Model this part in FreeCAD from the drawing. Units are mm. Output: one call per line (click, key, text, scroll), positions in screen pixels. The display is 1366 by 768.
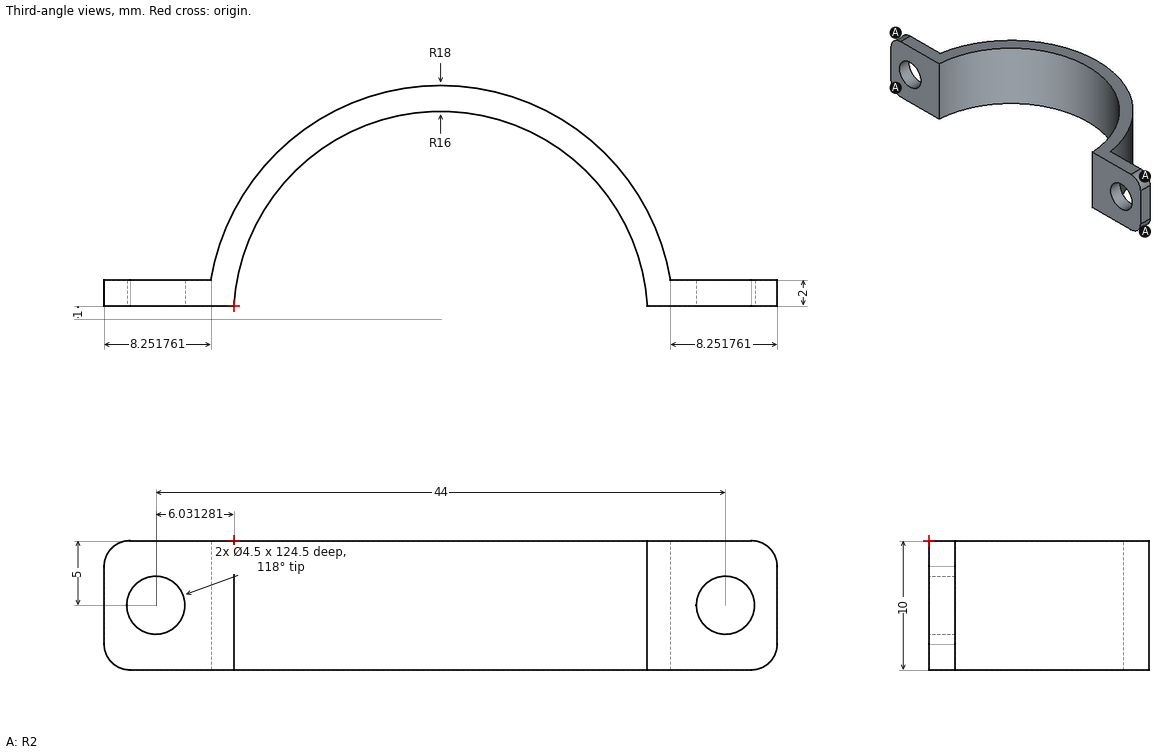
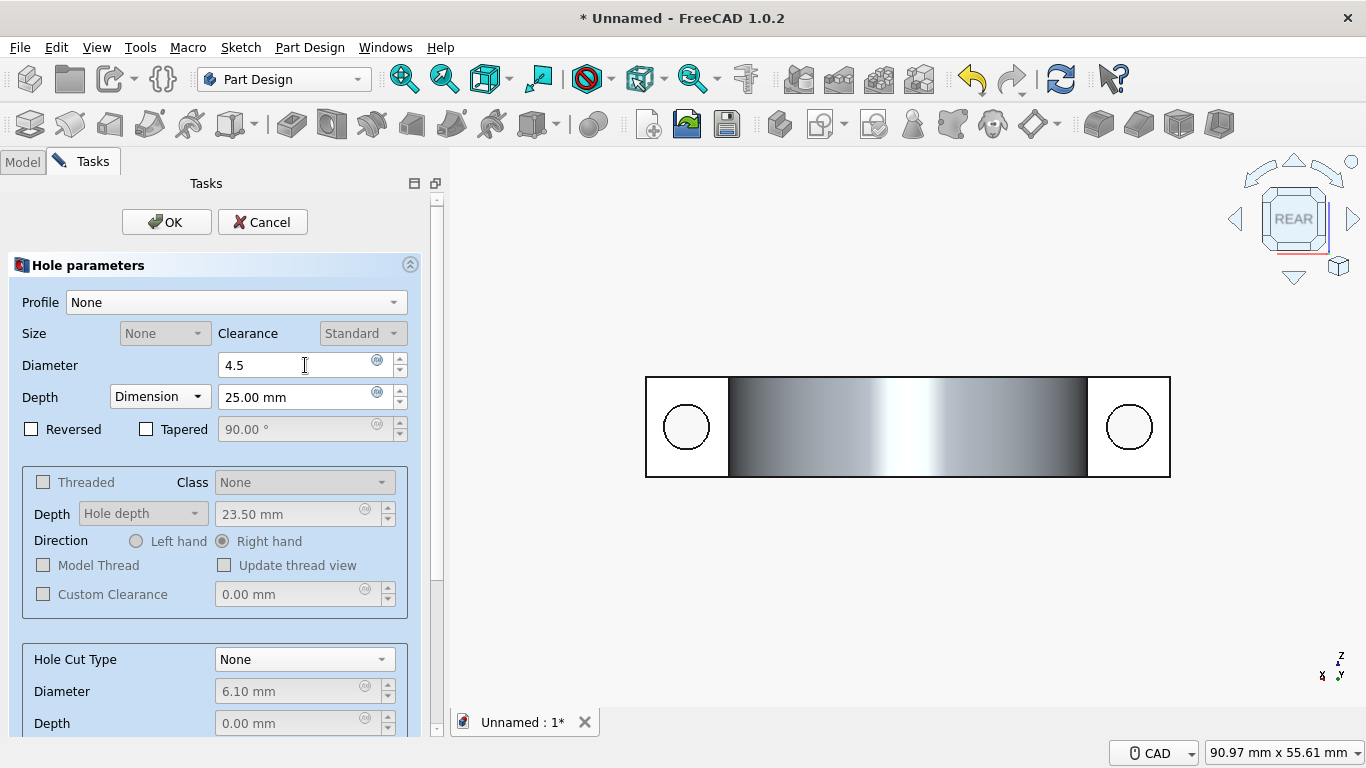
triple_click(305, 397)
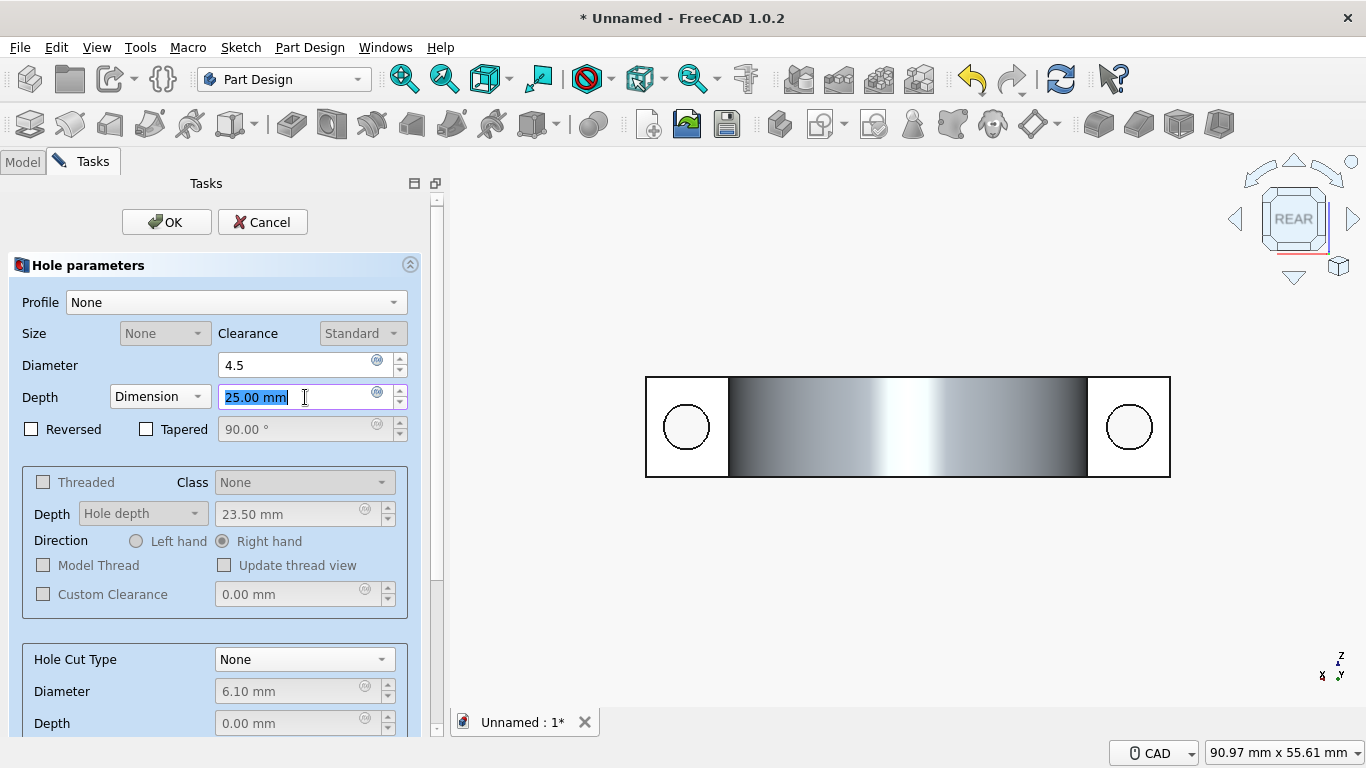
text(124.5)
key(Tab)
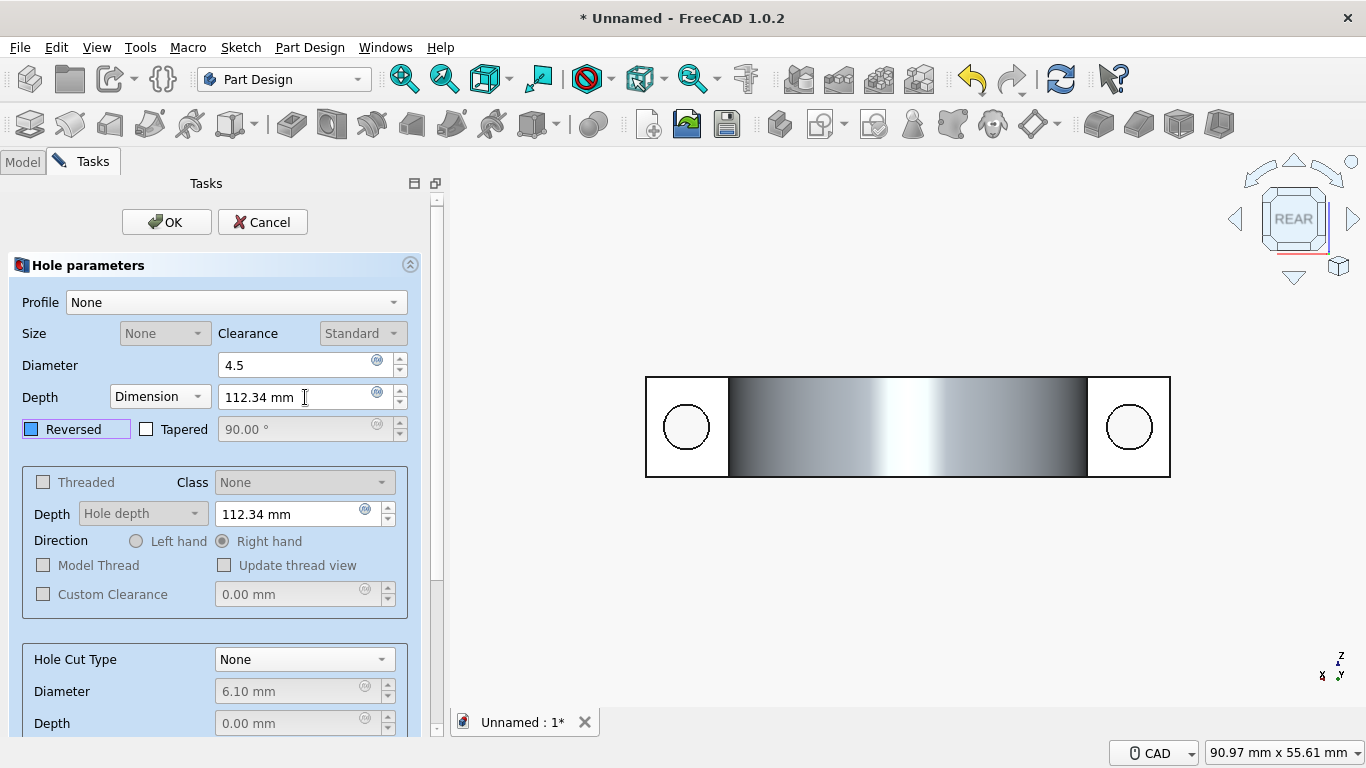
click(167, 222)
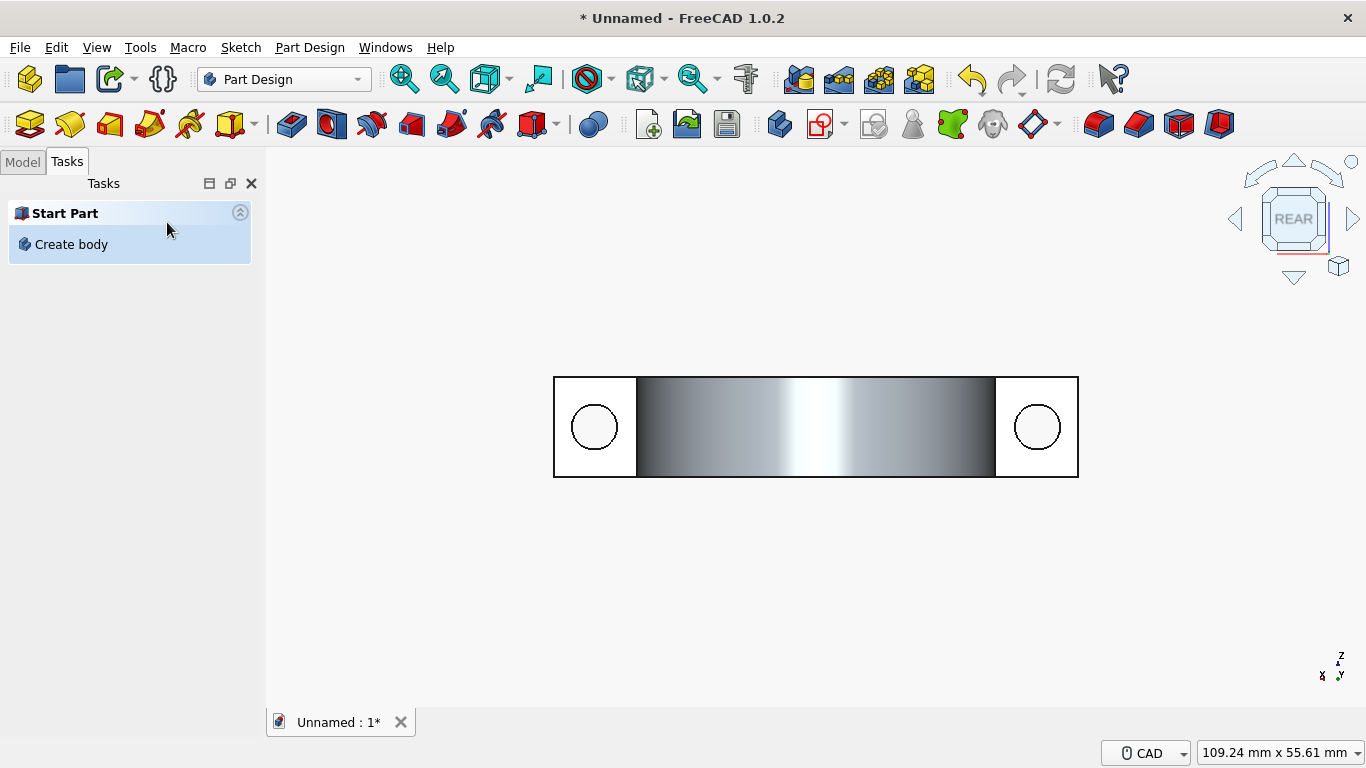
scroll(1078, 476, up, 4)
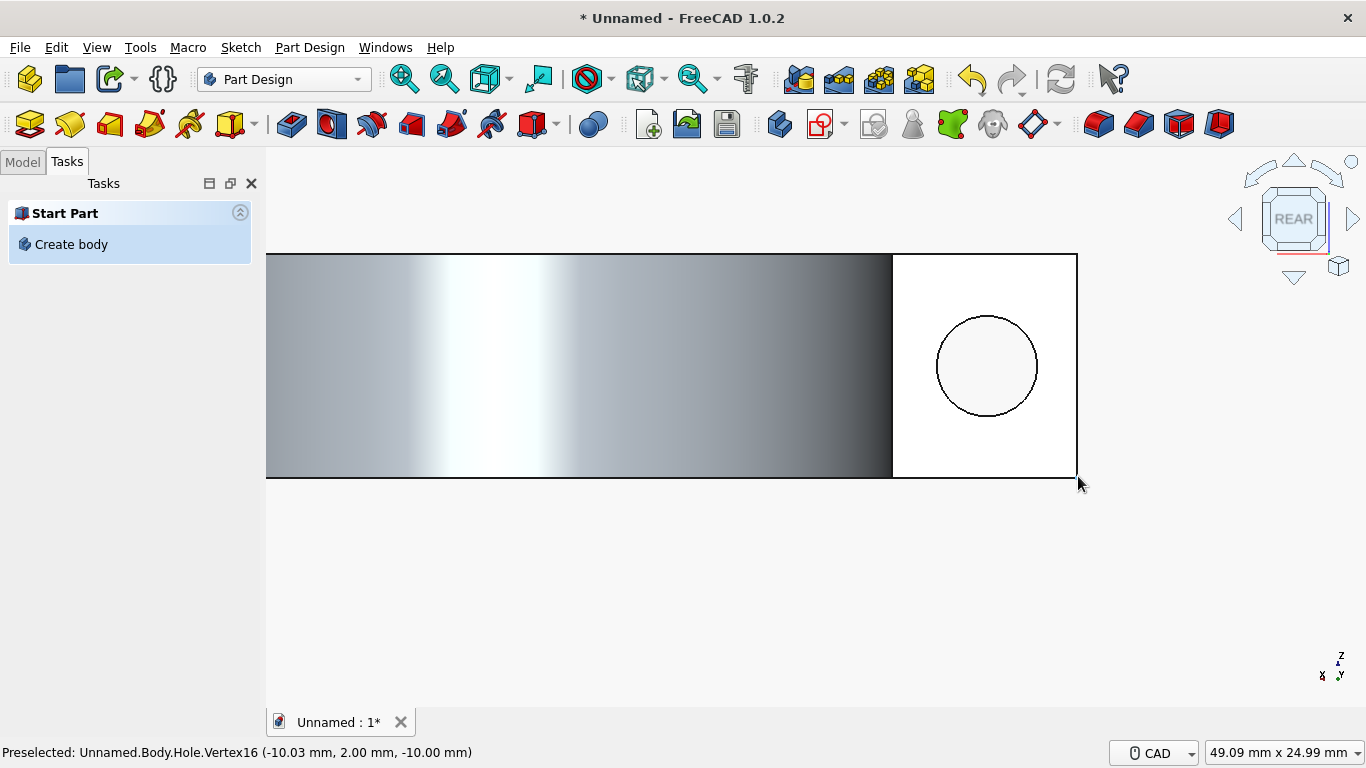
click(406, 80)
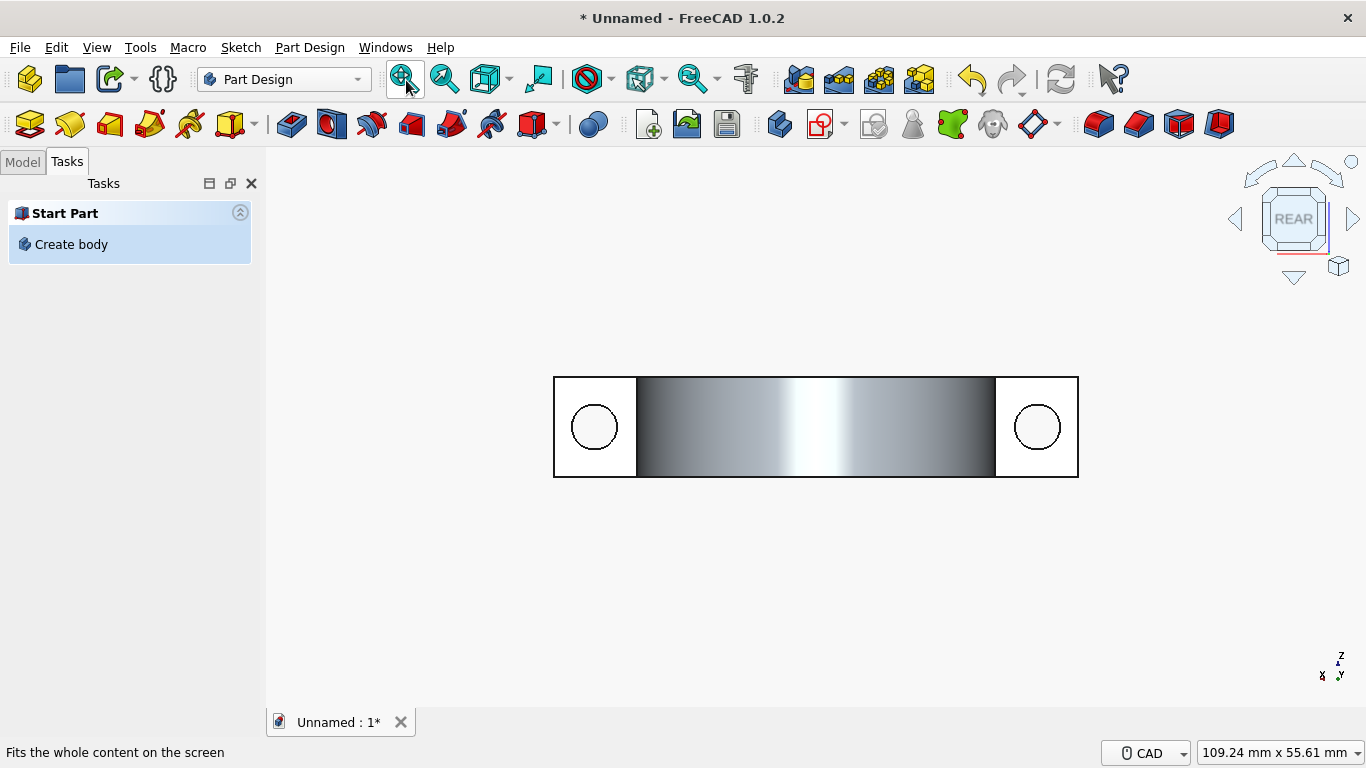
key(0)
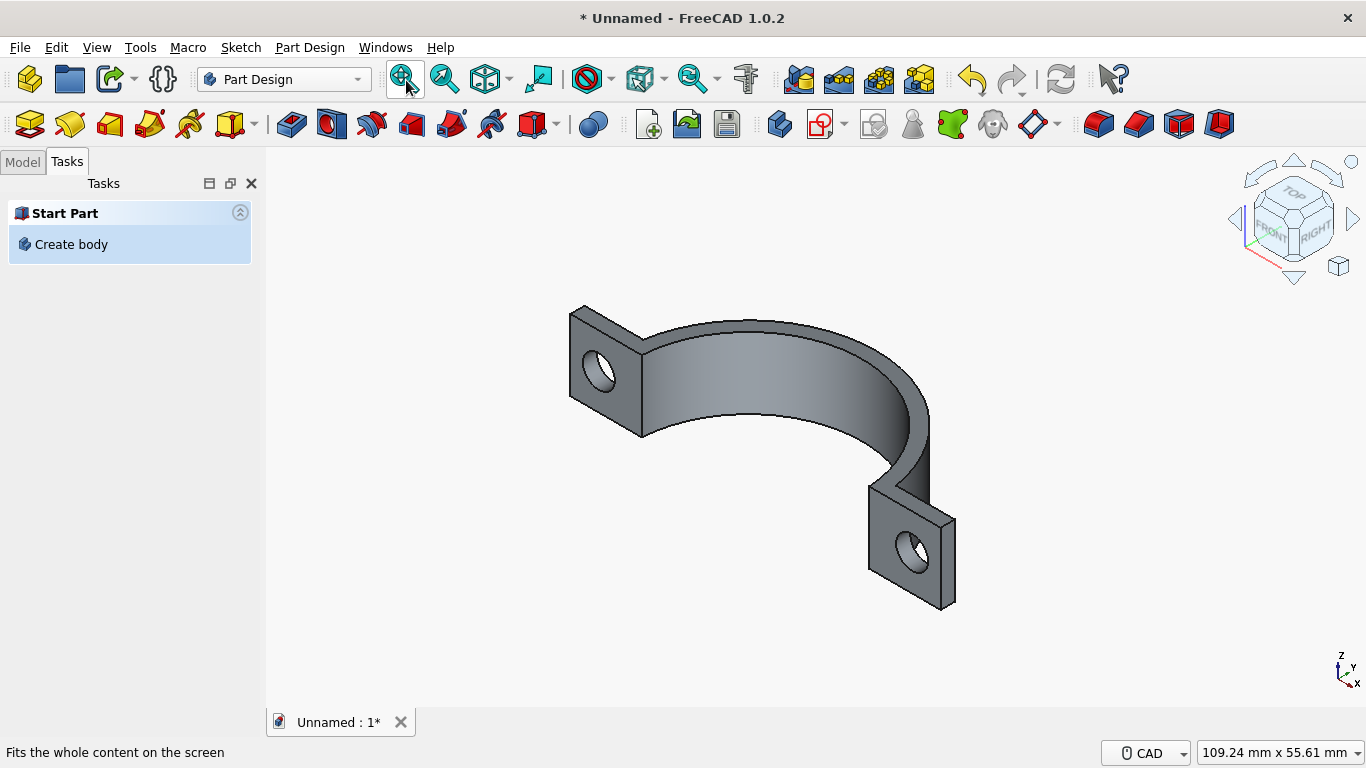
click(948, 523)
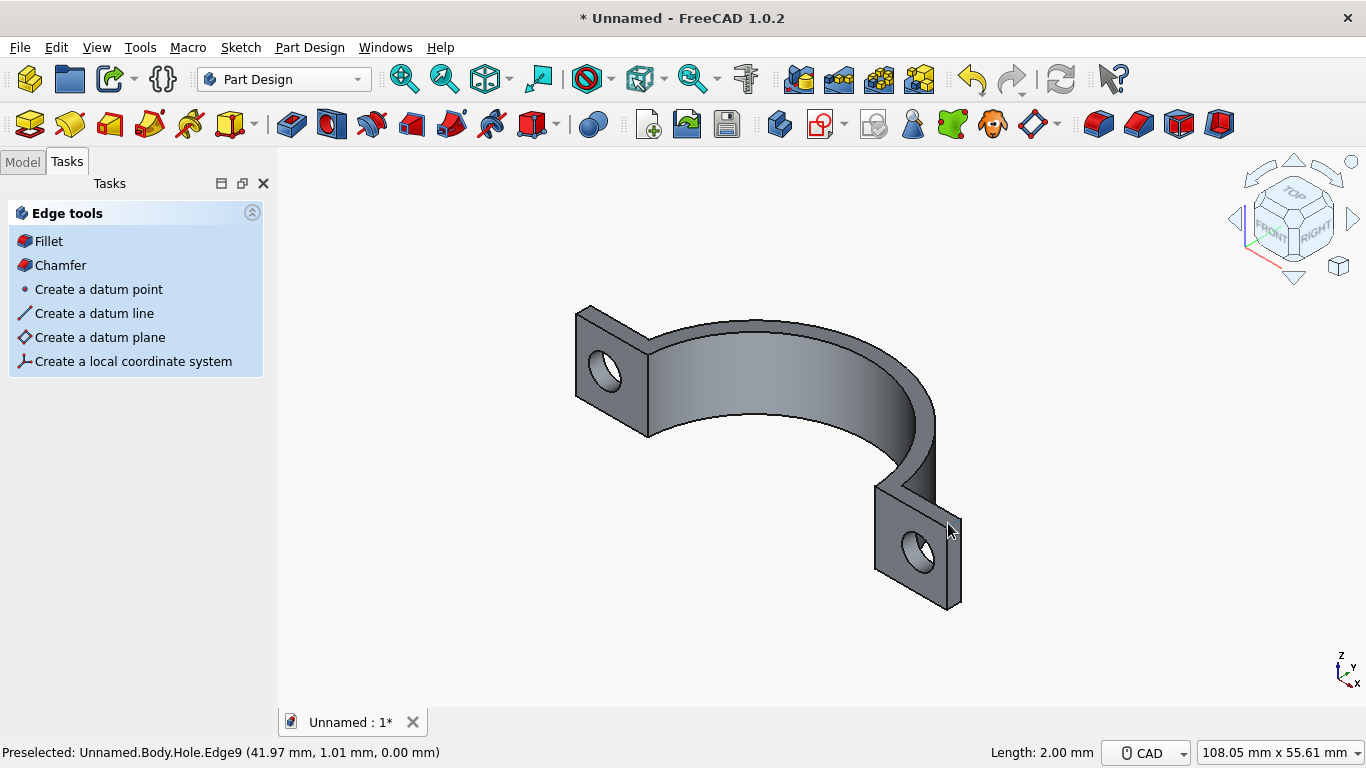
scroll(583, 391, up, 4)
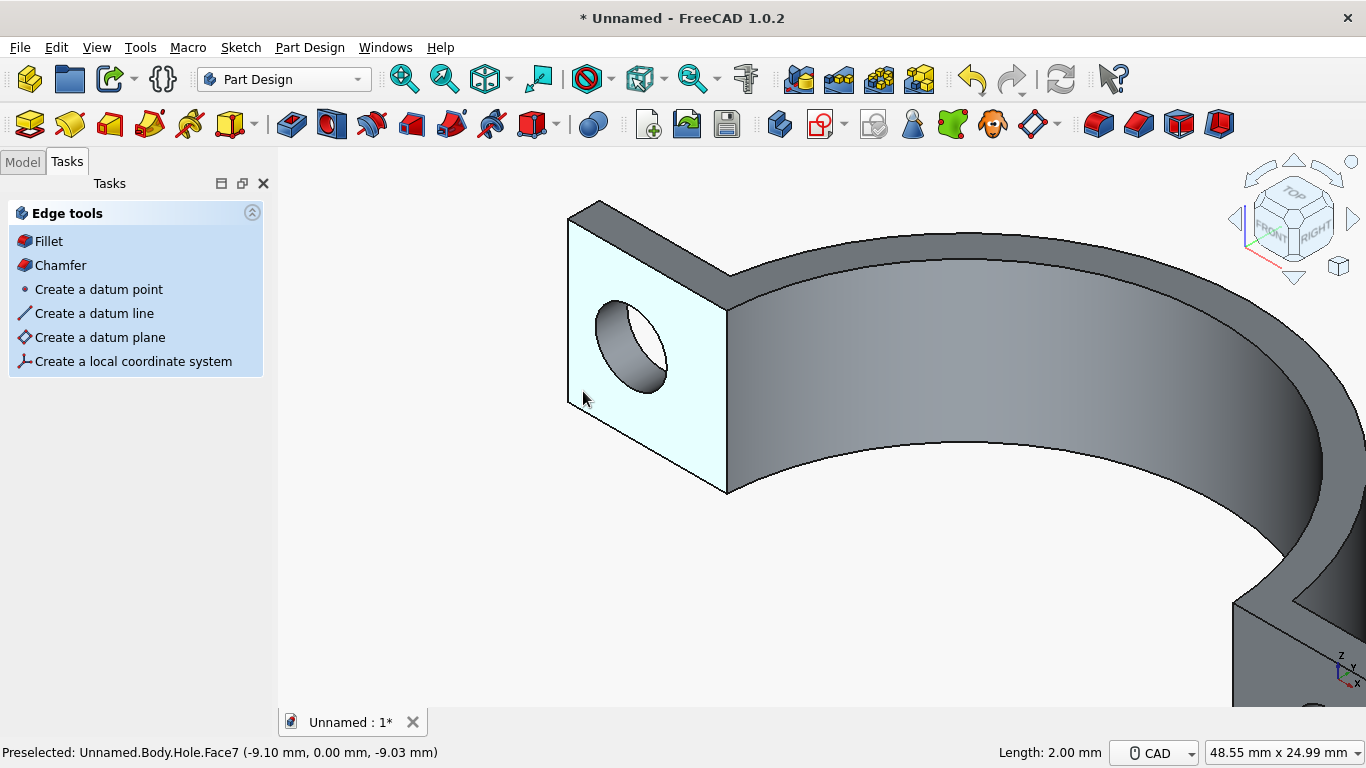
click(406, 80)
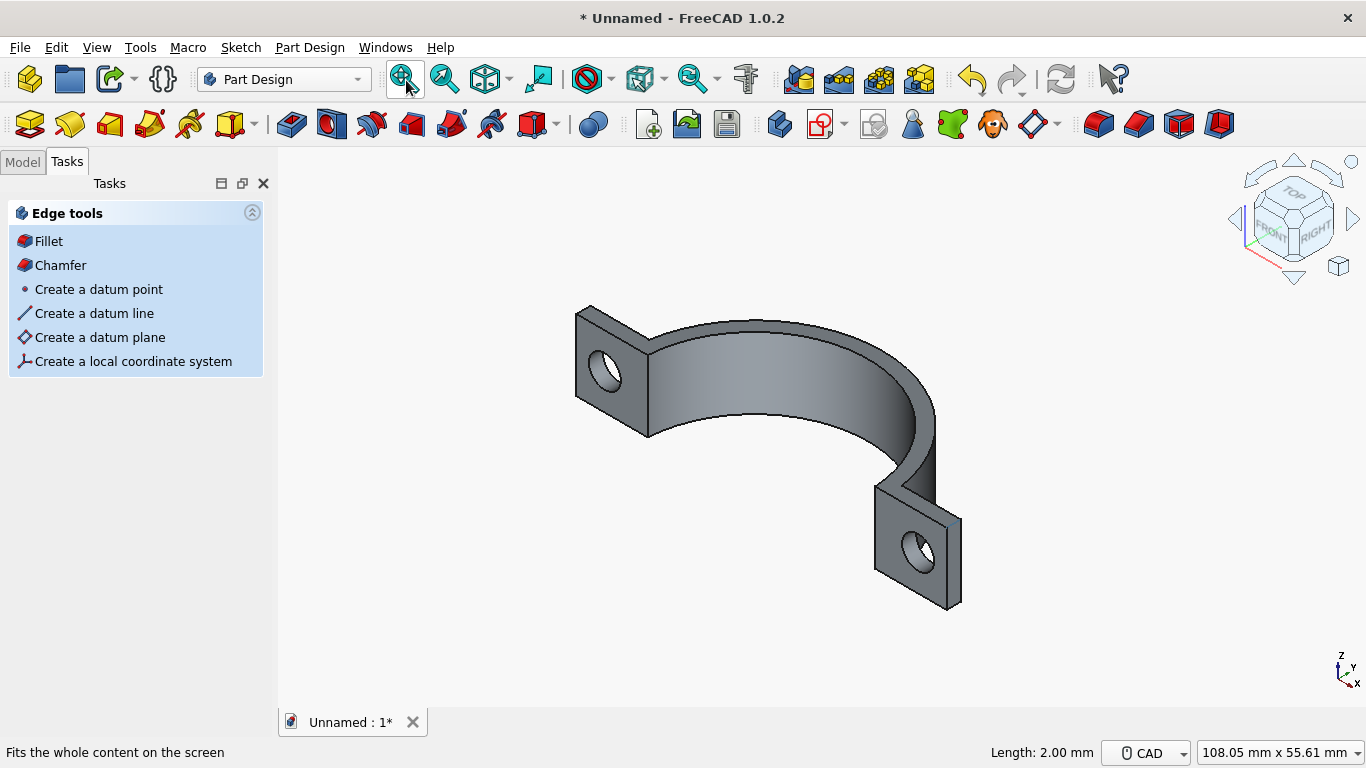
key(2)